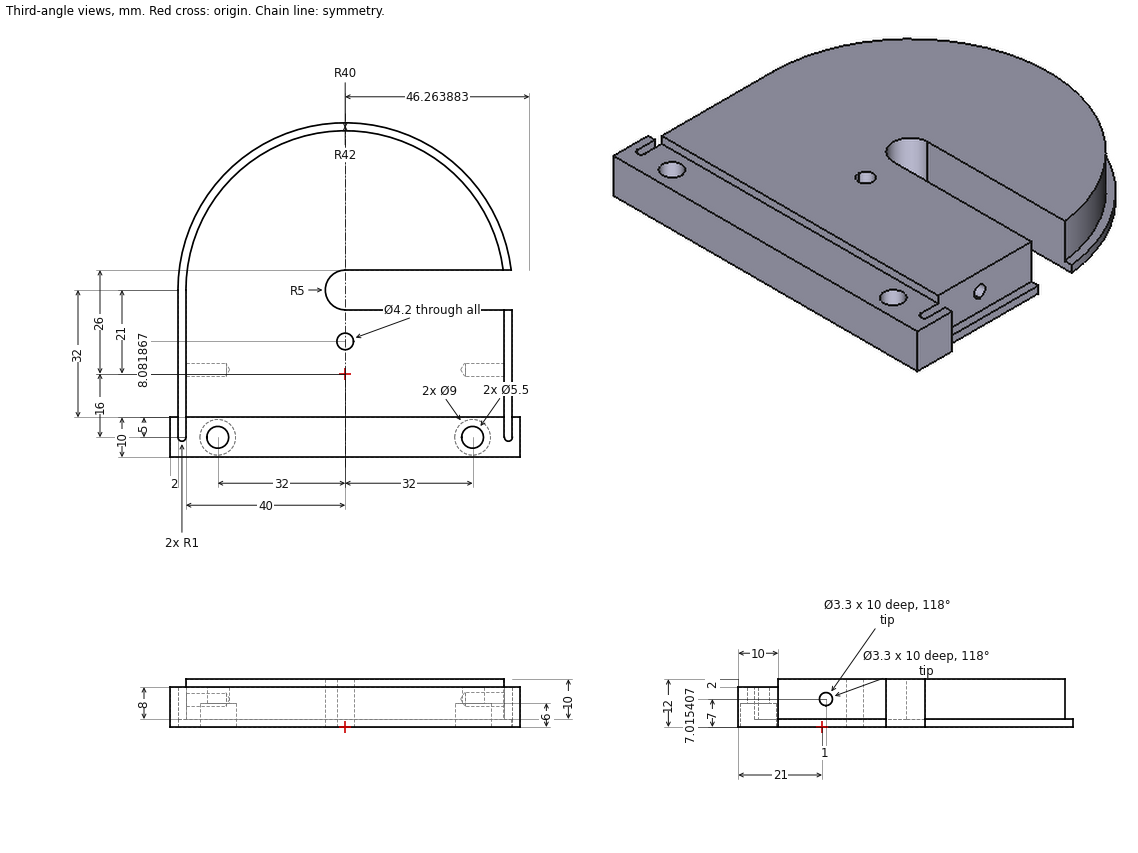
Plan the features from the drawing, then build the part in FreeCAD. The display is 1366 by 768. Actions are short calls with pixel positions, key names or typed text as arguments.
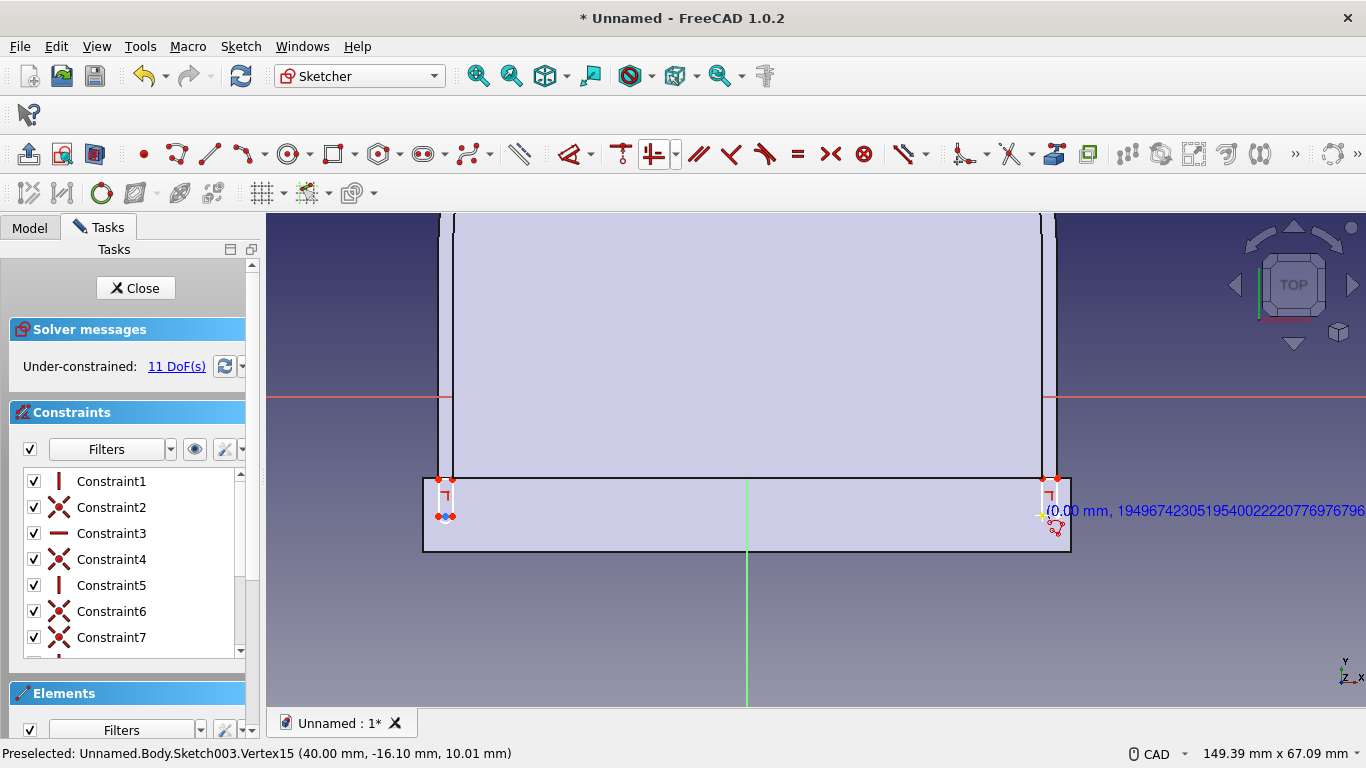
click(242, 154)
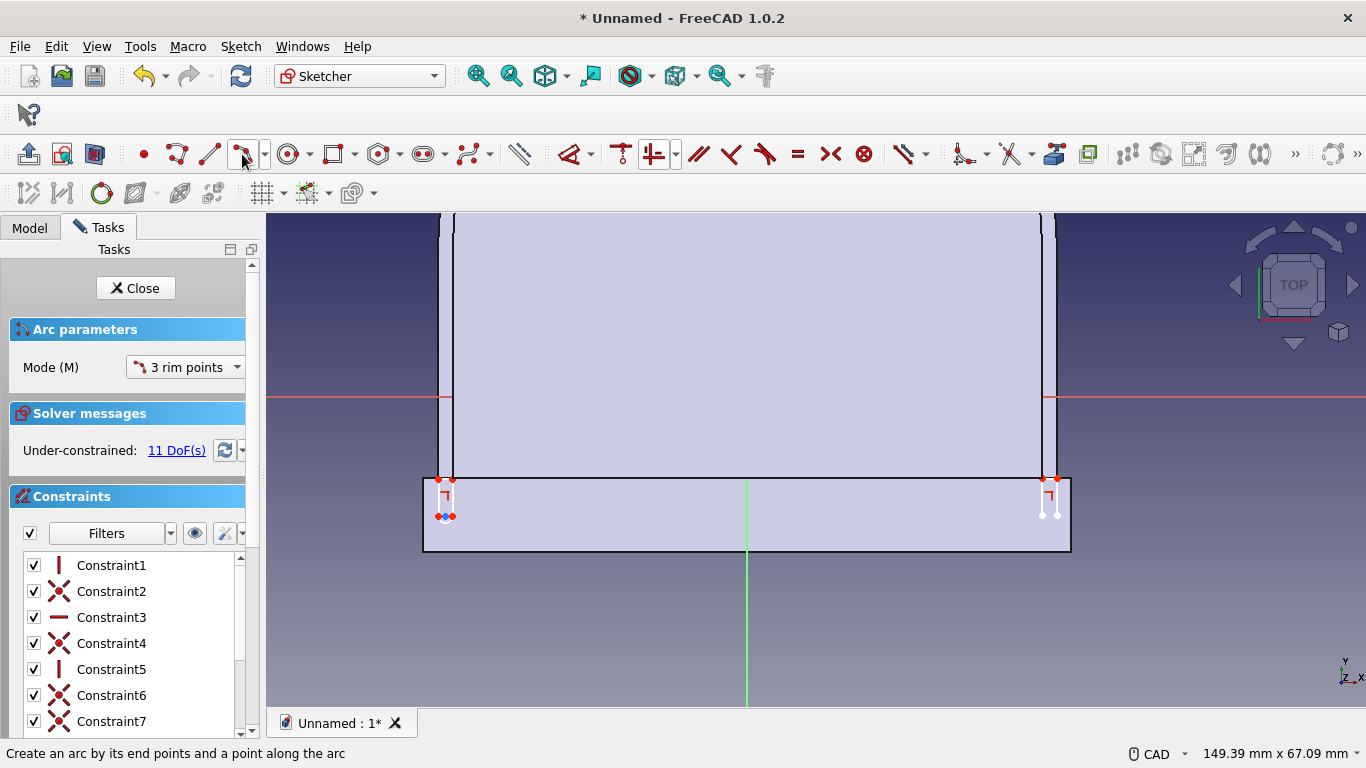
click(1042, 516)
click(1057, 516)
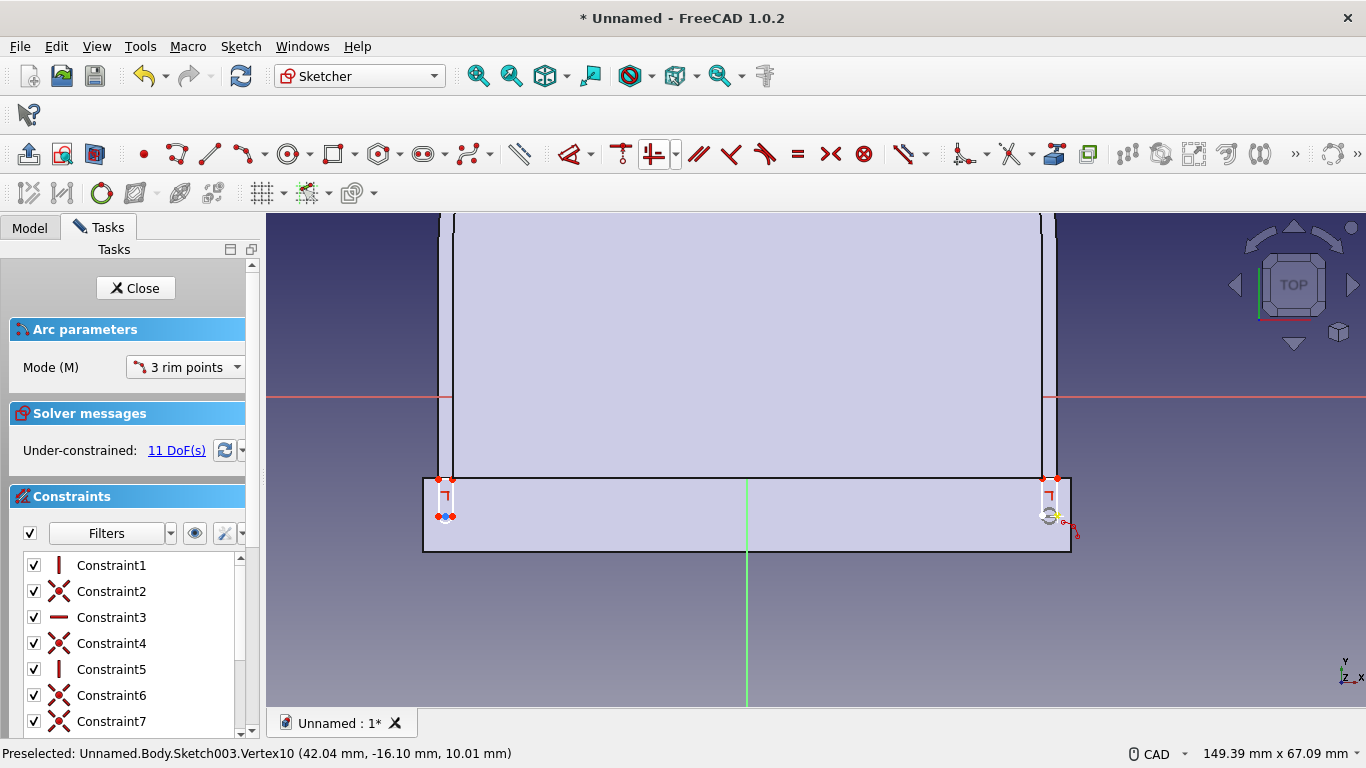
scroll(1049, 523, up, 4)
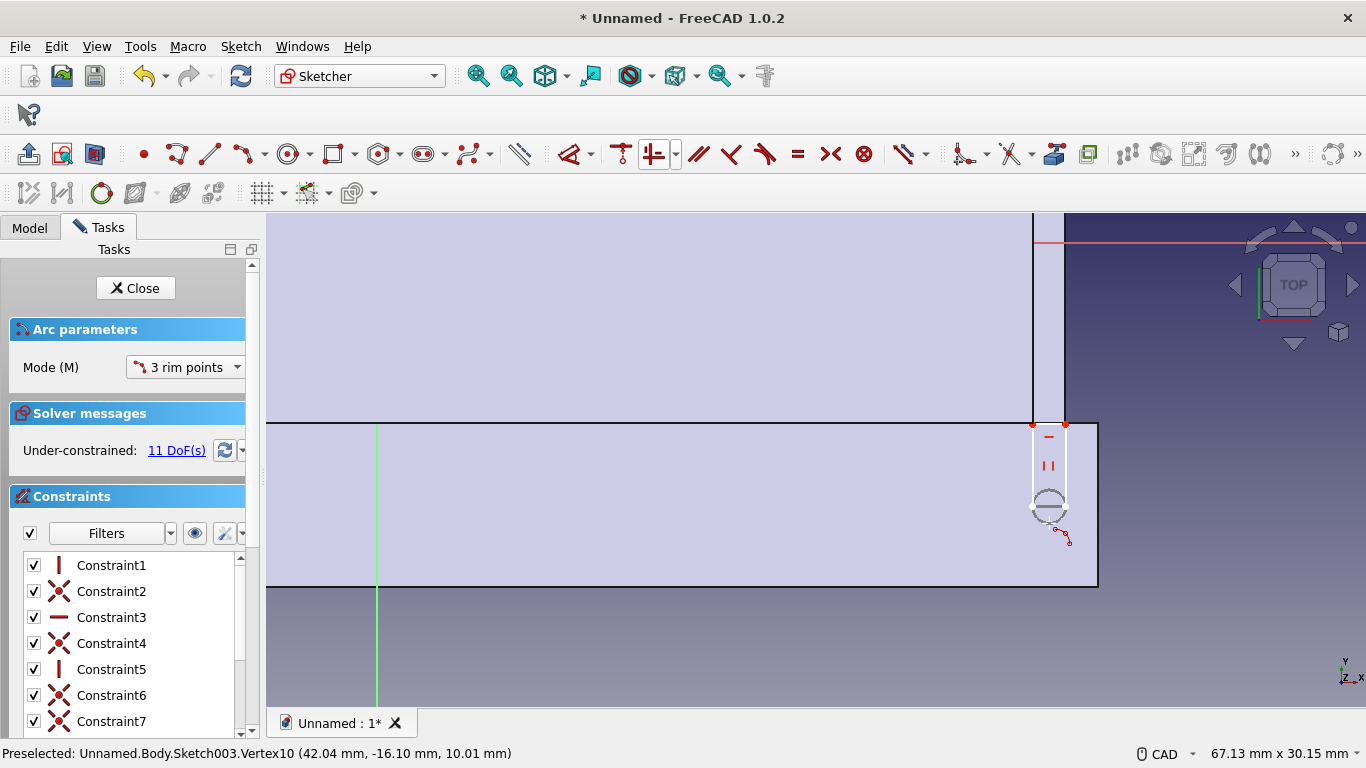
click(1049, 521)
key(Escape)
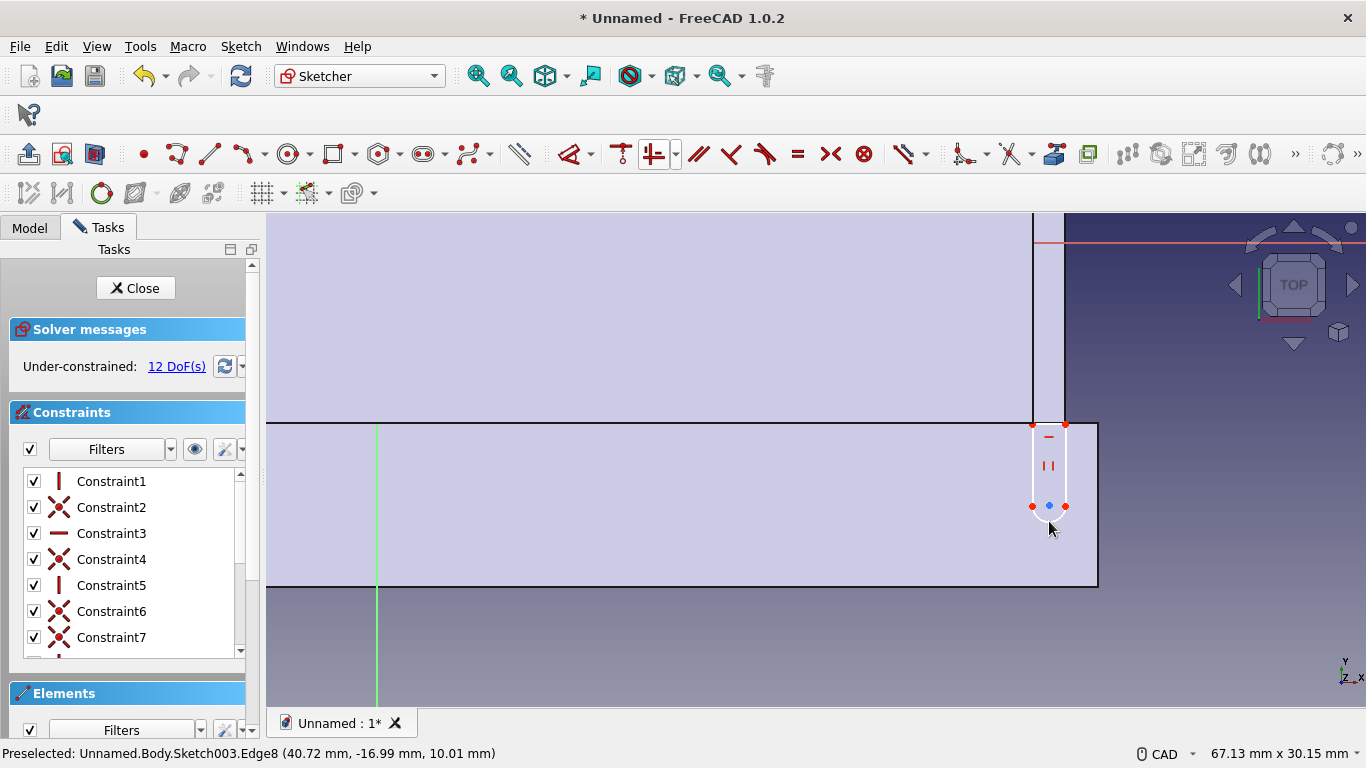
scroll(1050, 524, down, 4)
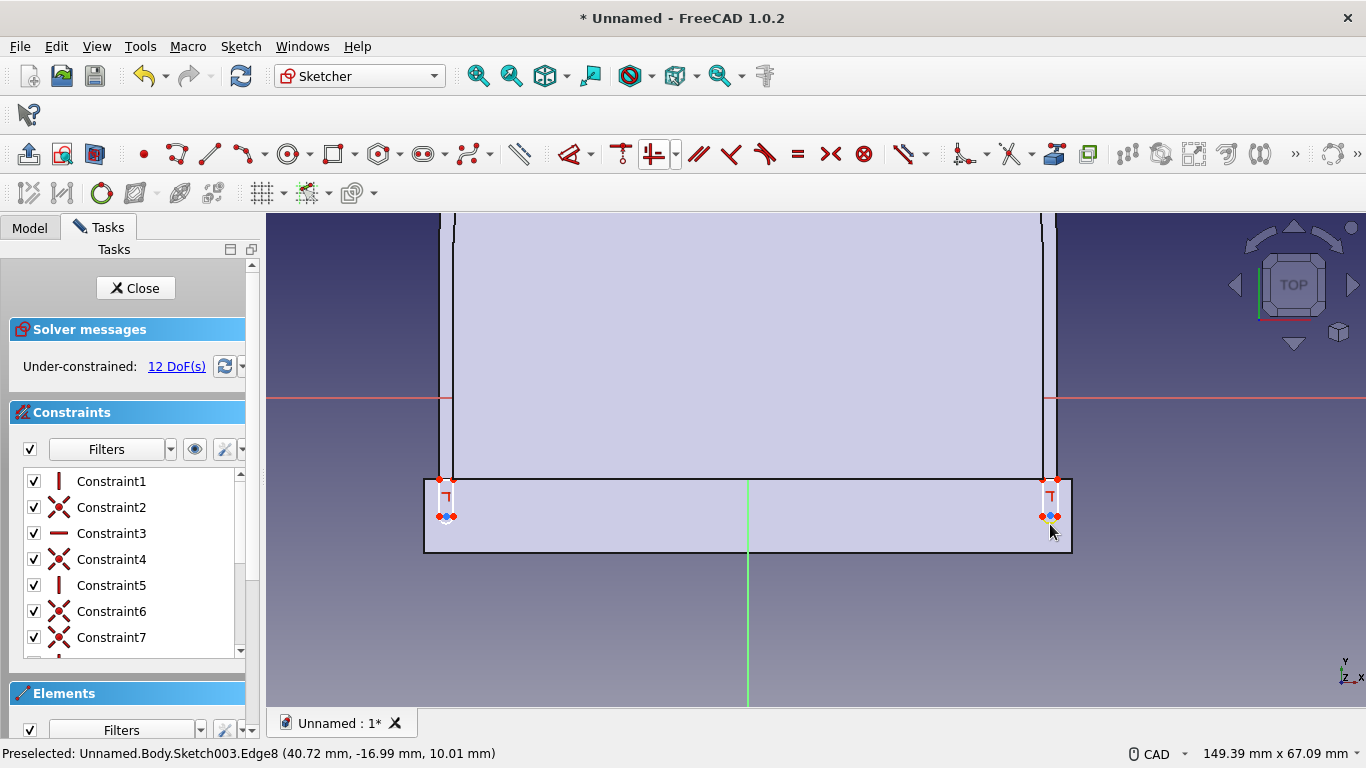
scroll(453, 506, up, 2)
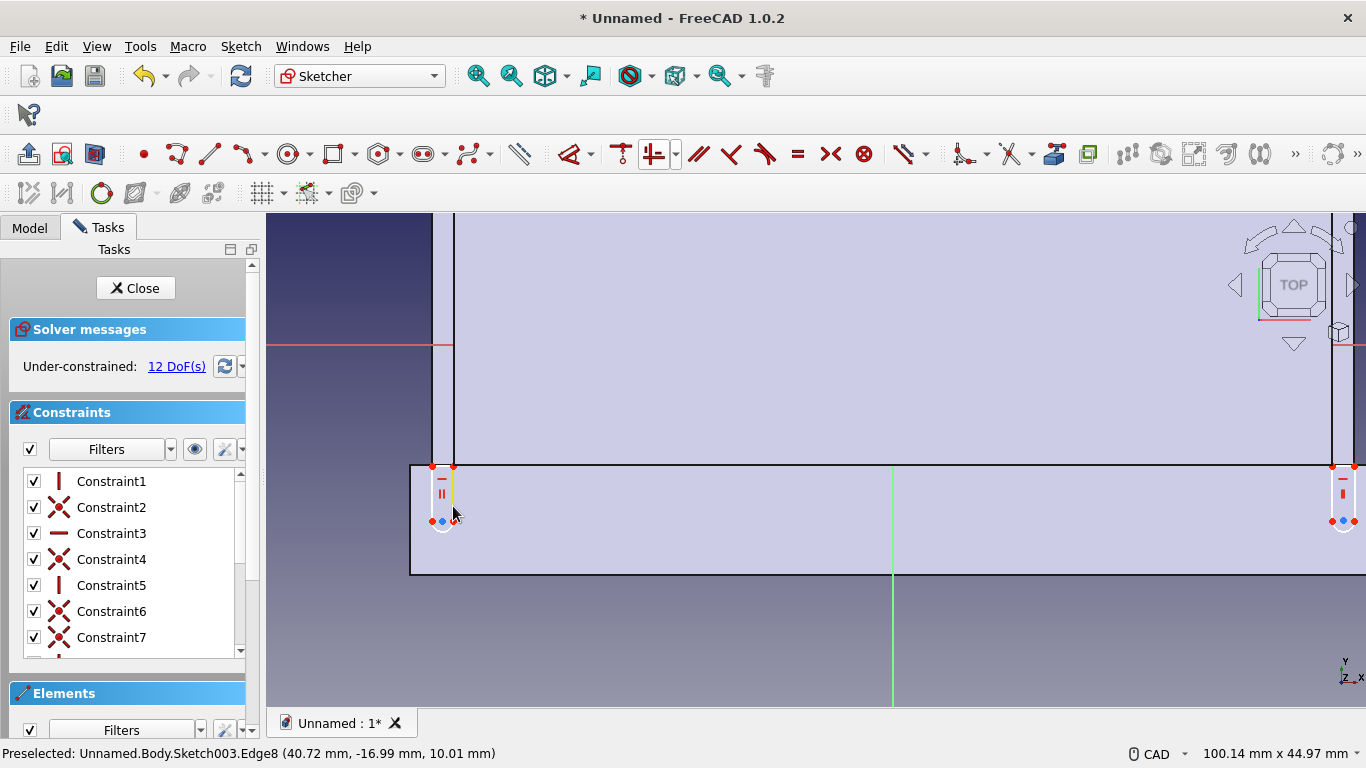
click(453, 505)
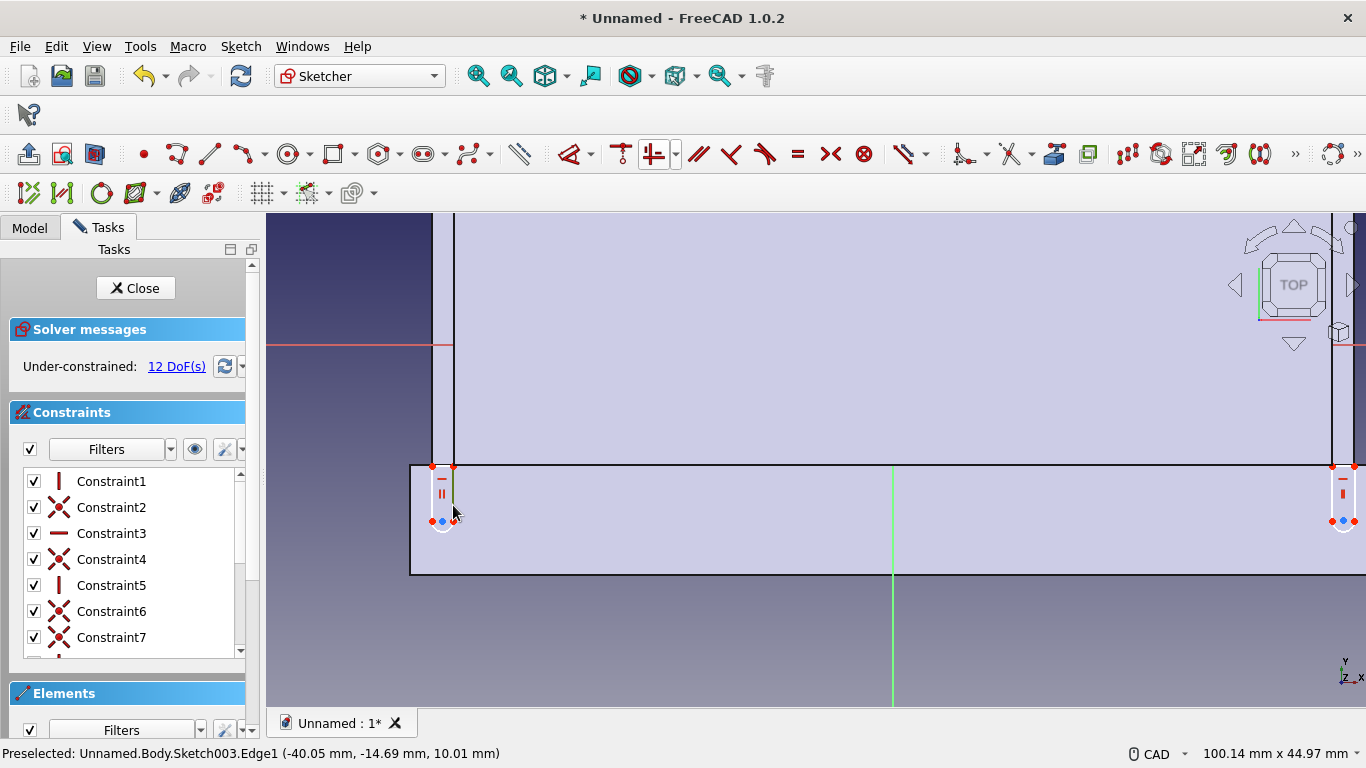
scroll(437, 530, up, 2)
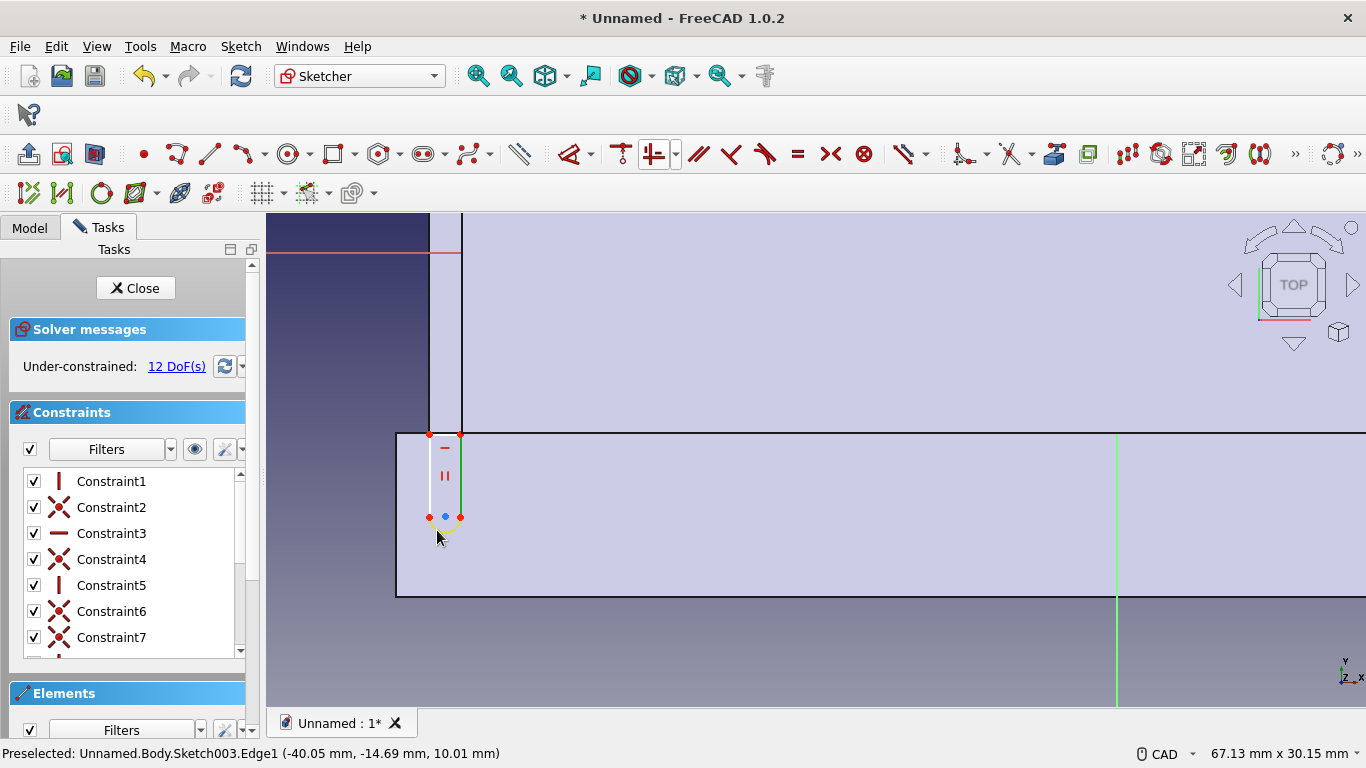
click(436, 530)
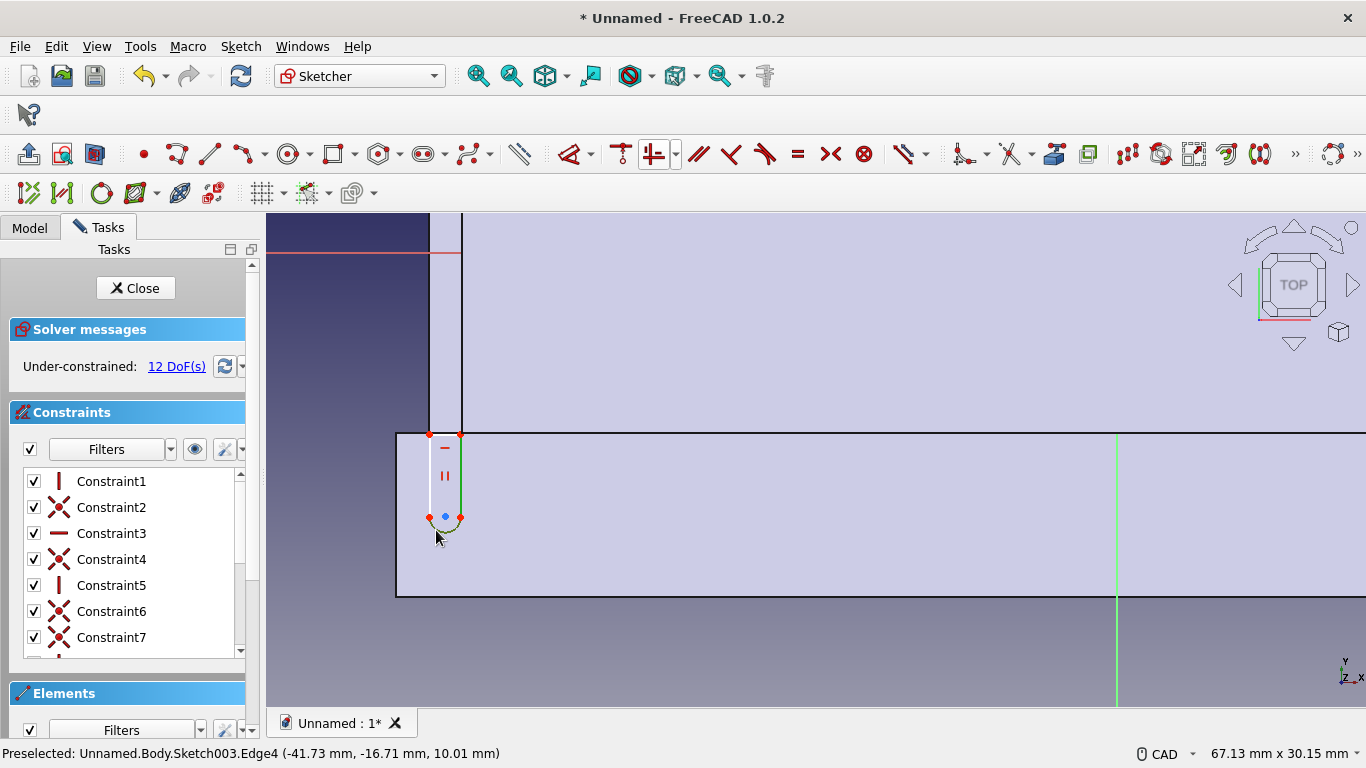
click(765, 154)